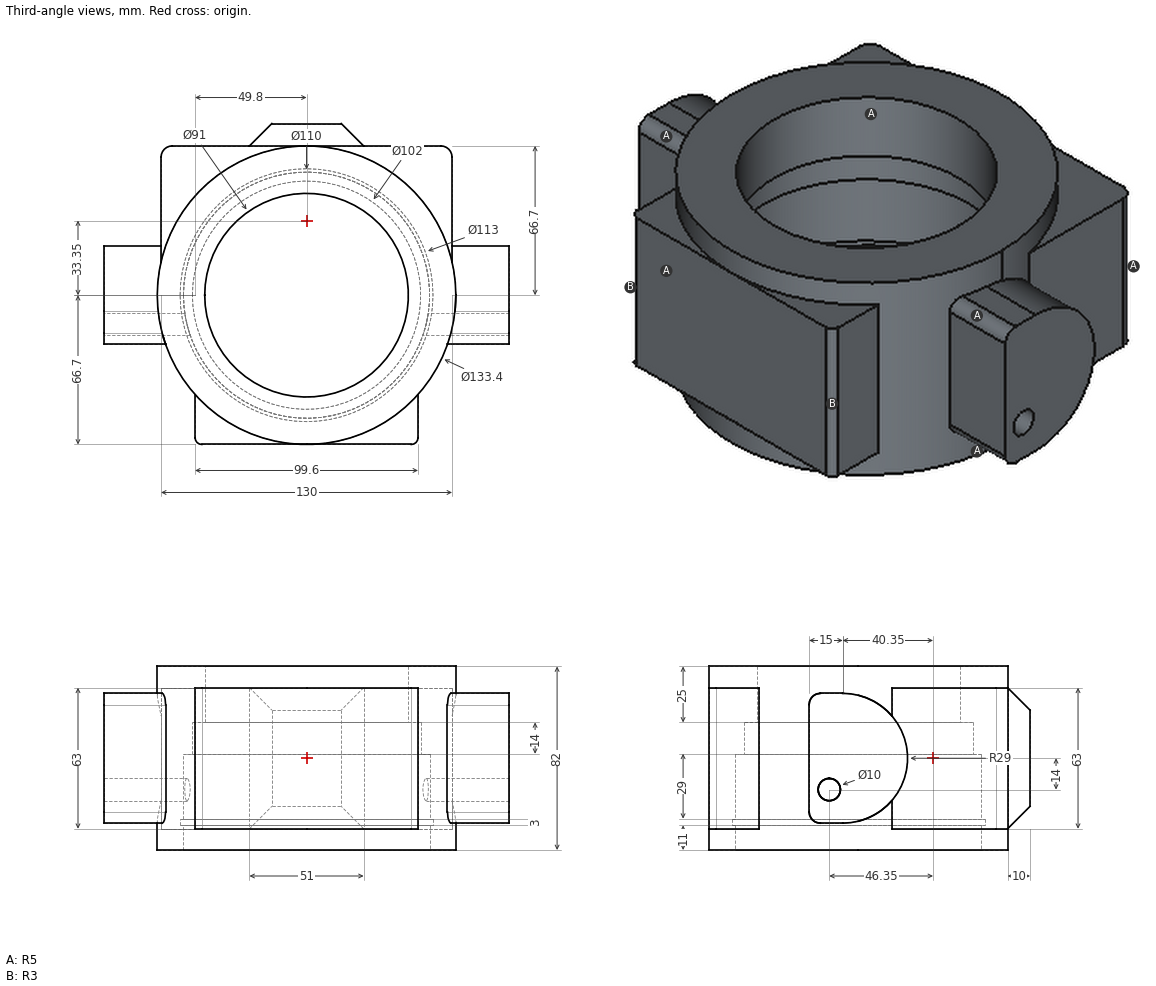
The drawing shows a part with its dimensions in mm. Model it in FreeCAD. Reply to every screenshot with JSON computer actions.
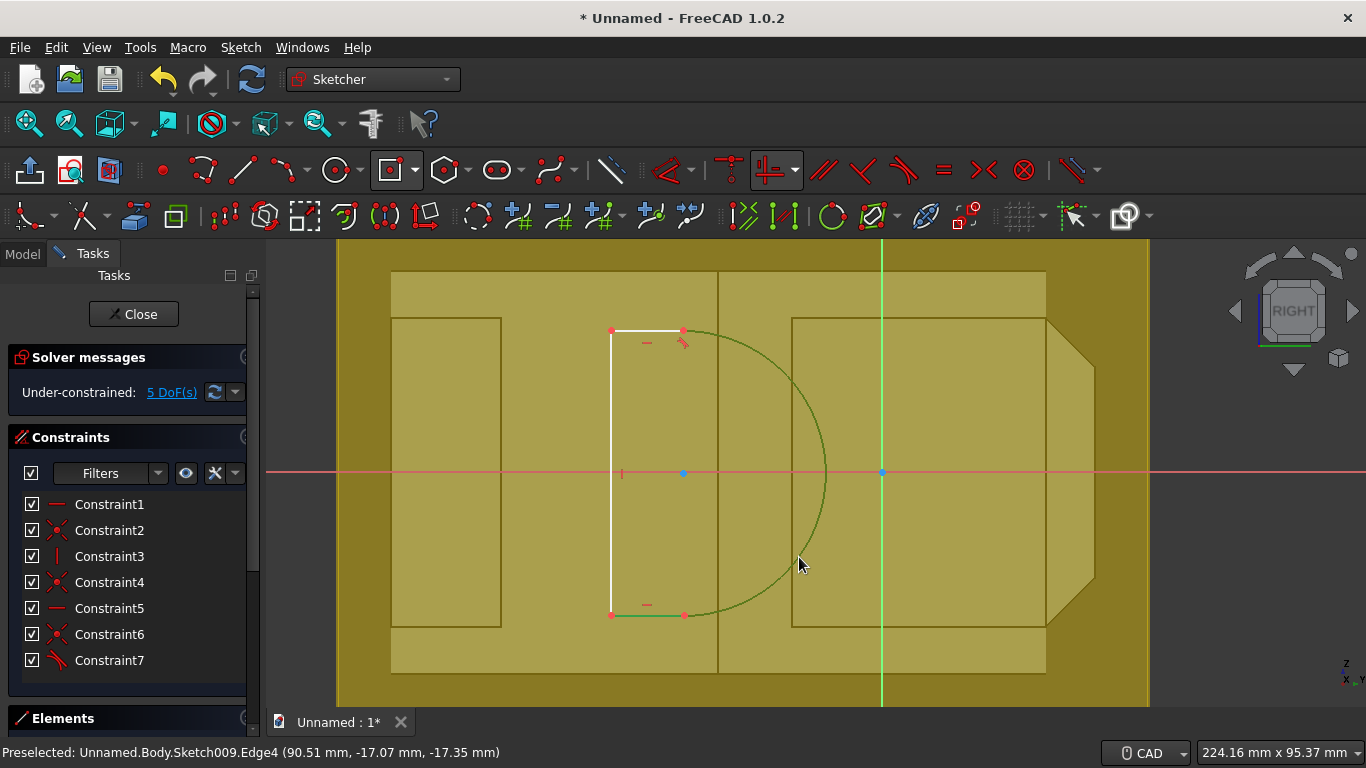
{"action": "key", "text": "t"}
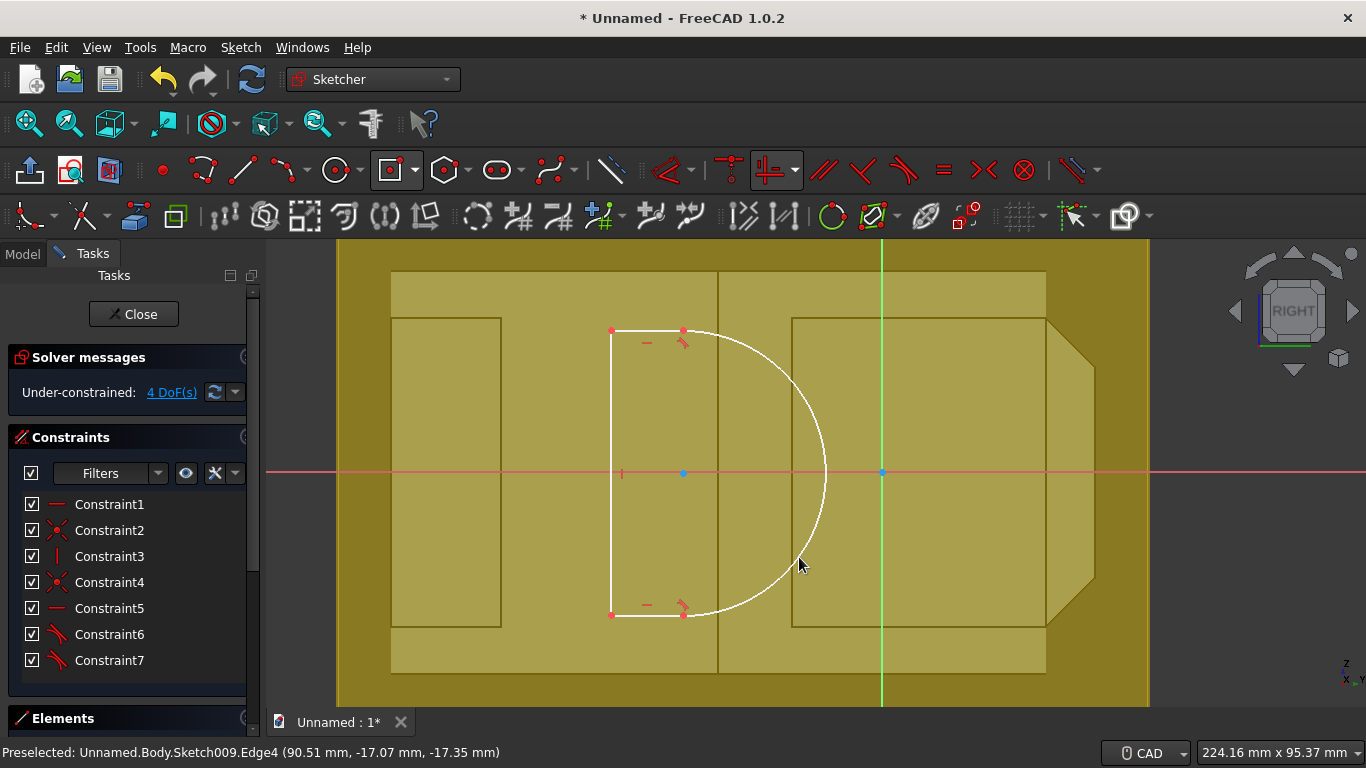
{"action": "left_click", "coordinate": [683, 473]}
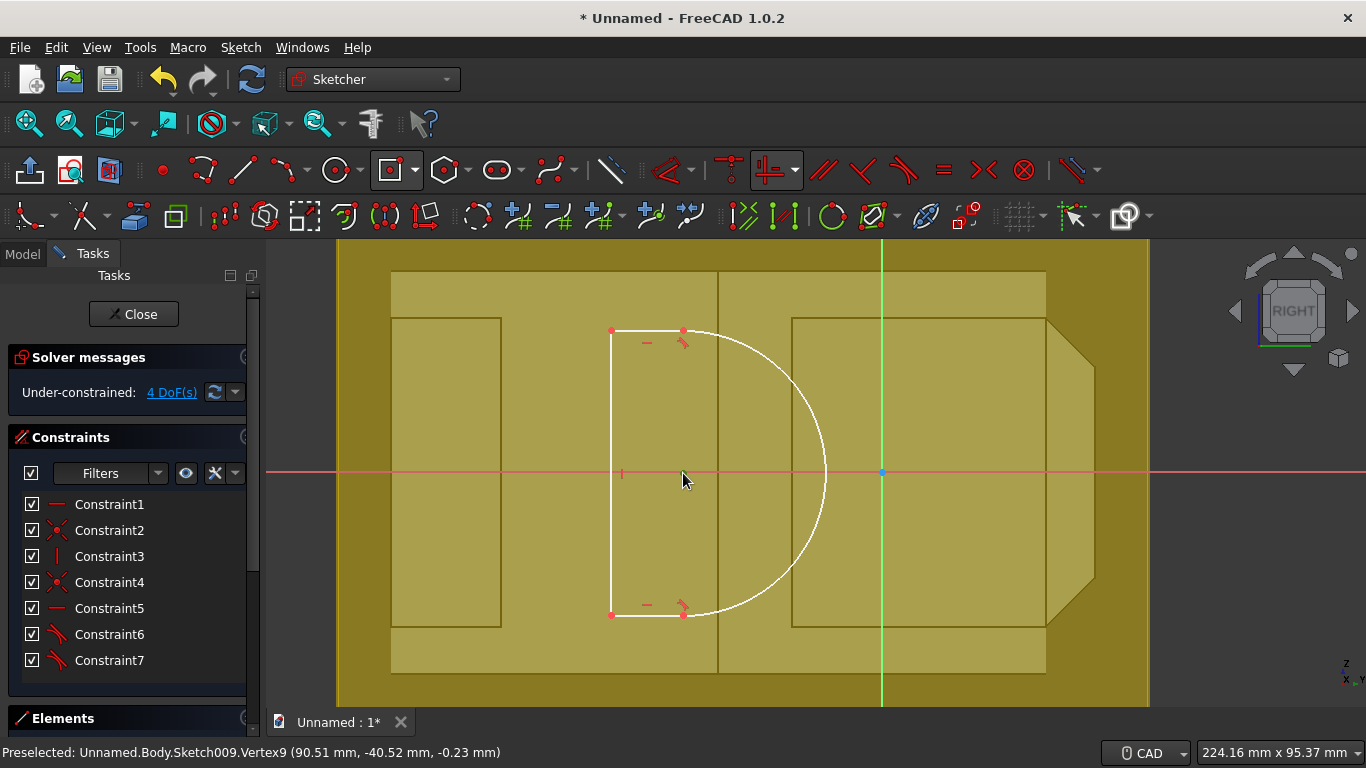
{"action": "left_click", "coordinate": [359, 472]}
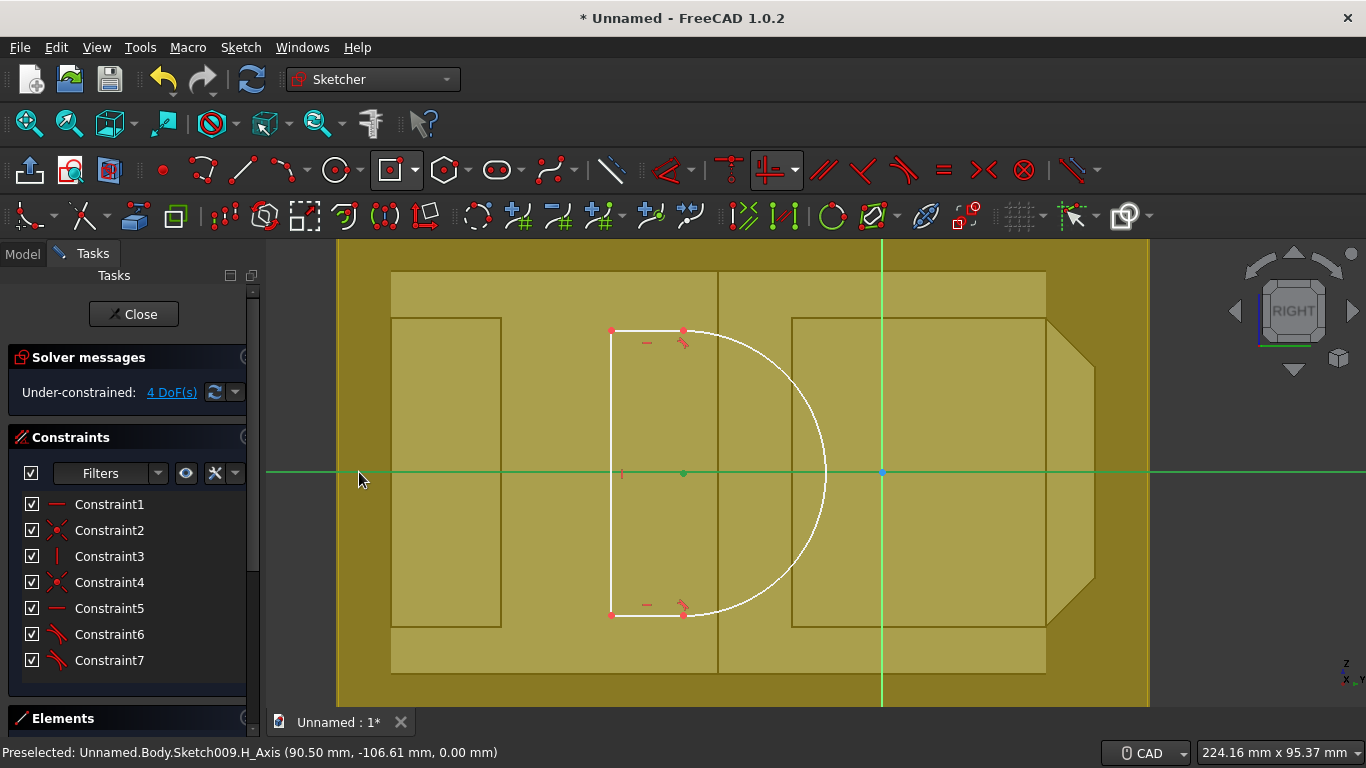
{"action": "key", "text": "c"}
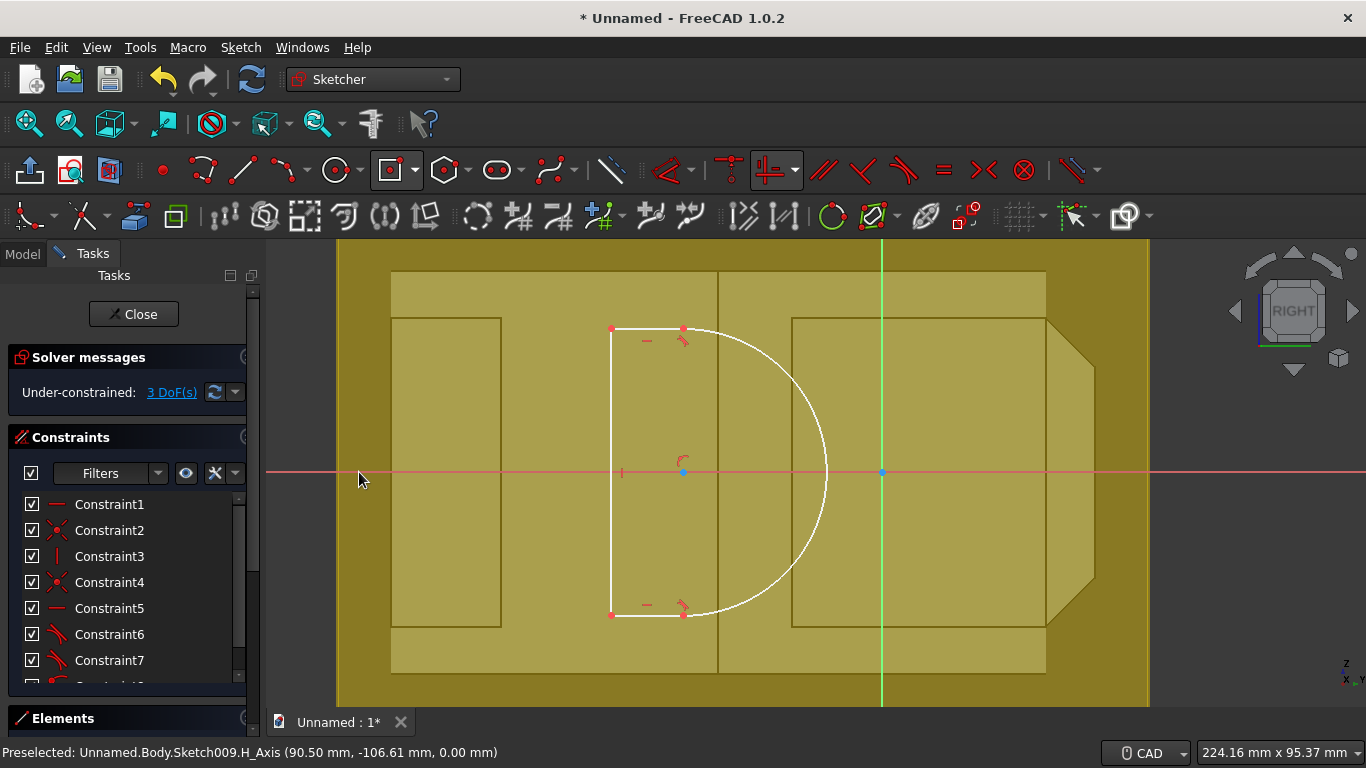
{"action": "key", "text": "d"}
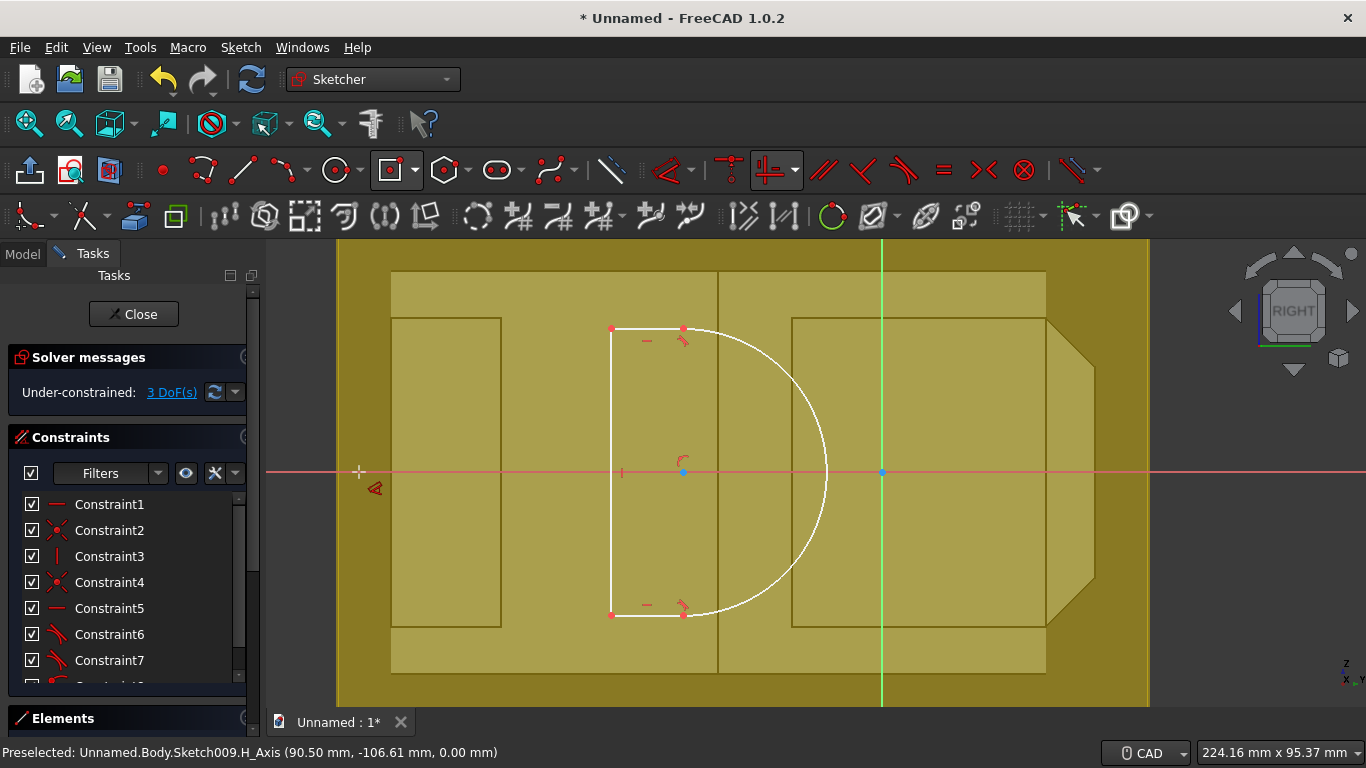
{"action": "left_click", "coordinate": [799, 557]}
{"action": "left_click", "coordinate": [825, 576]}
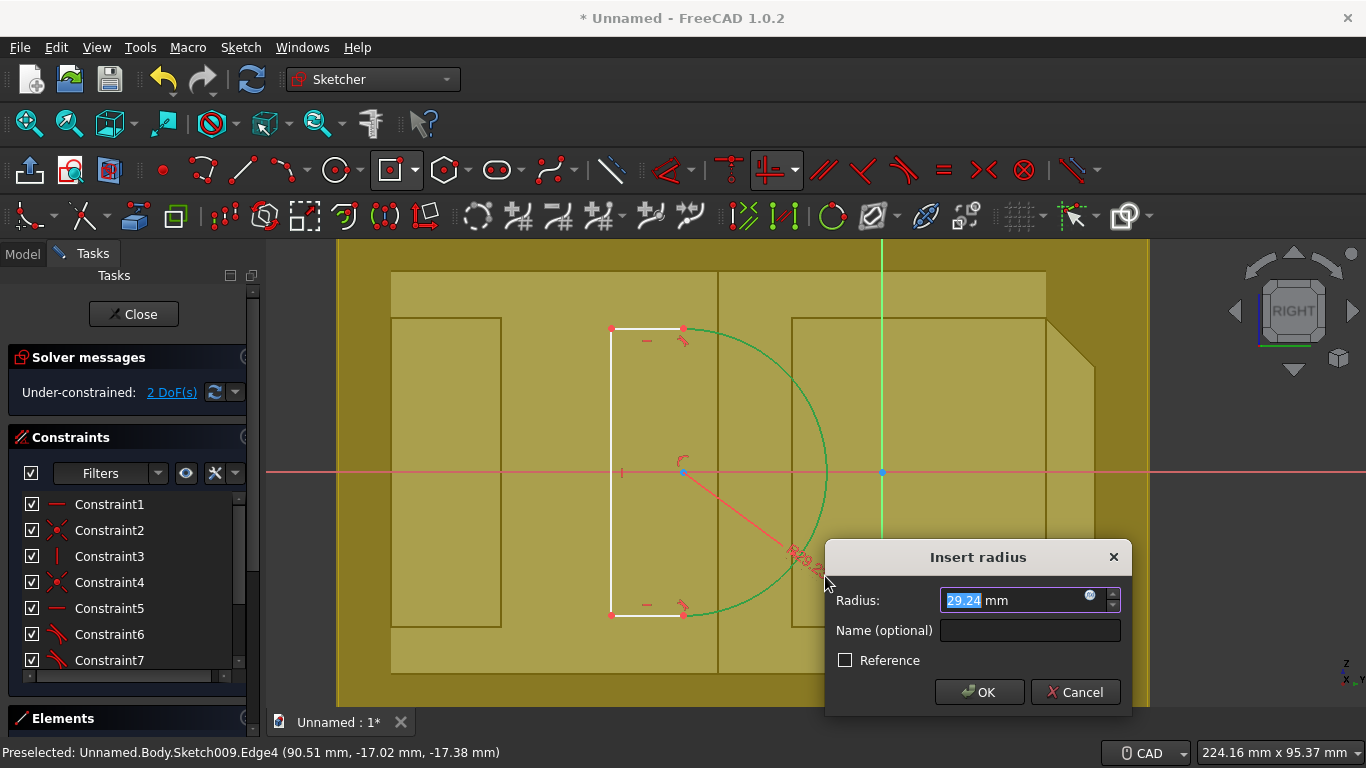
{"action": "type", "text": "29"}
{"action": "key", "text": "Return"}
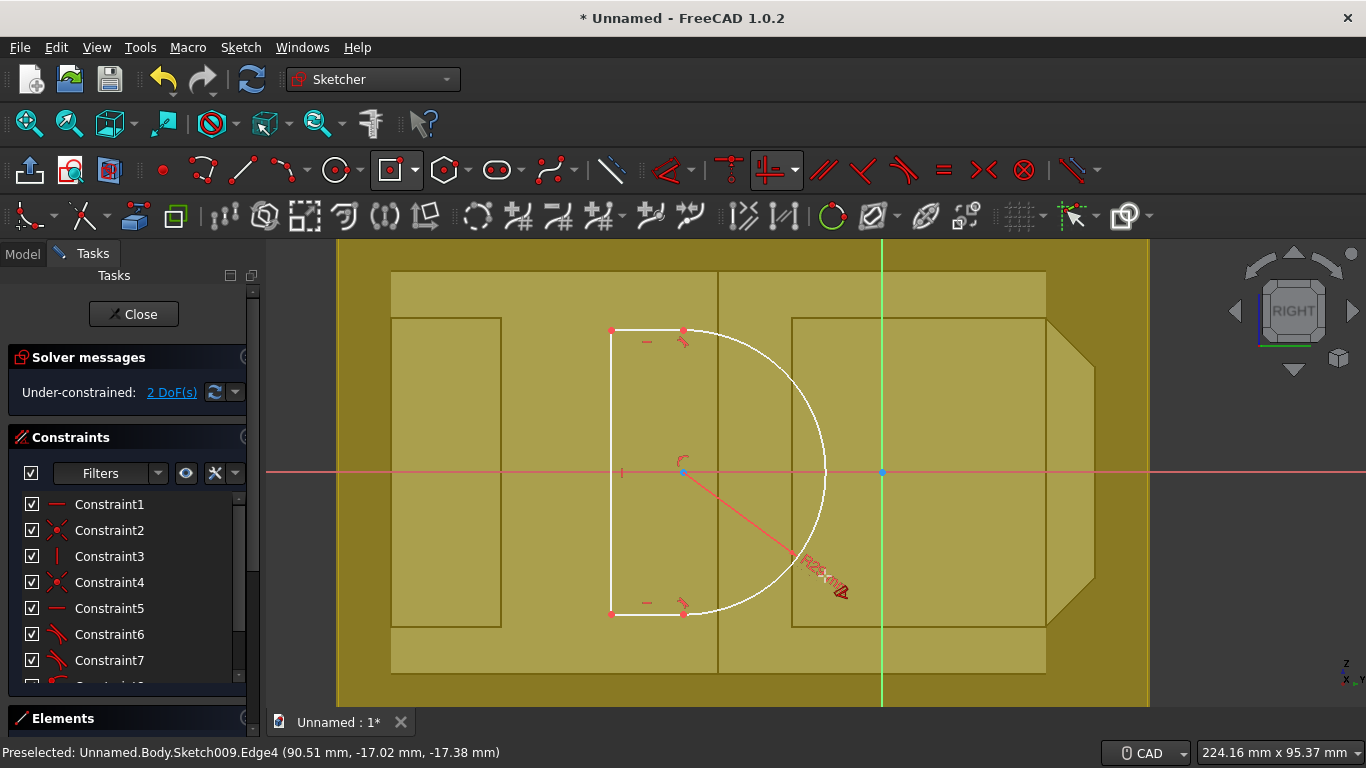
{"action": "left_click", "coordinate": [662, 330]}
{"action": "left_click", "coordinate": [647, 296]}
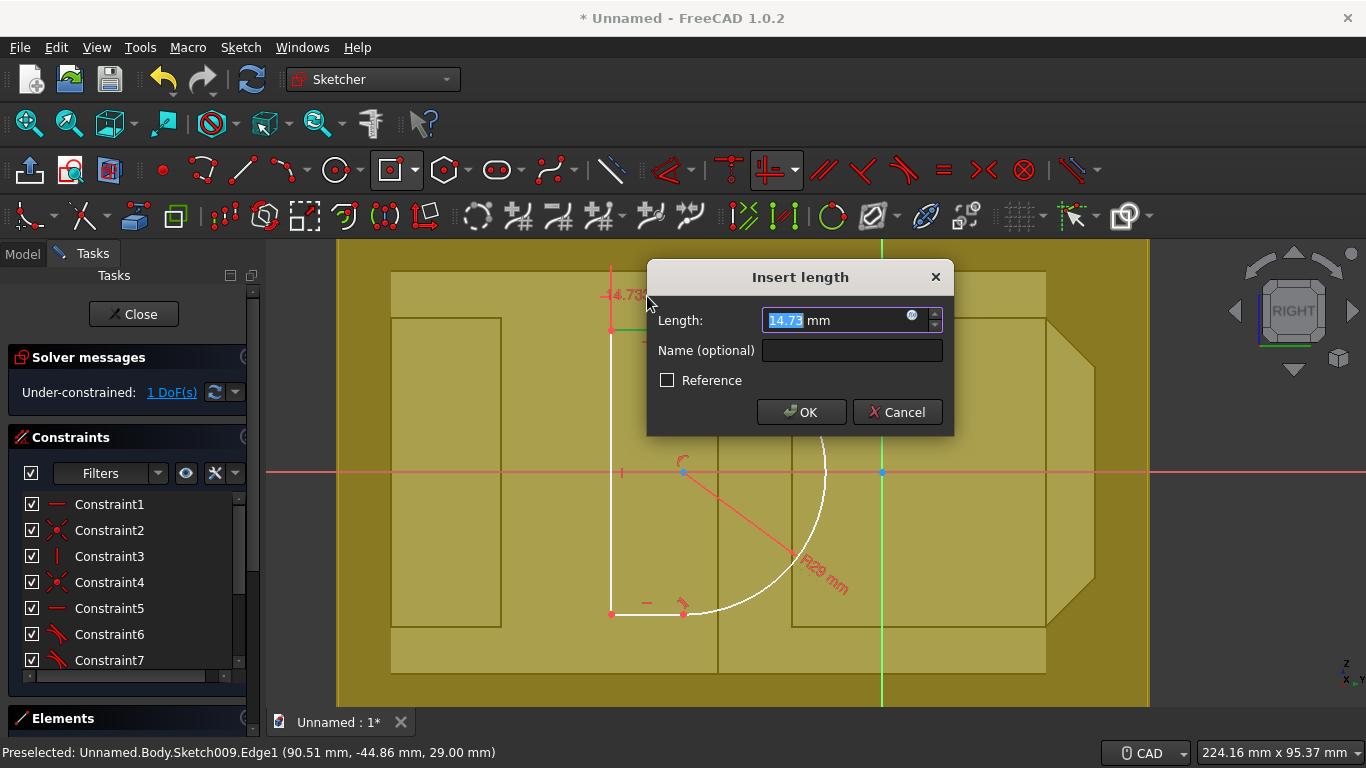
{"action": "type", "text": "15"}
{"action": "key", "text": "Return"}